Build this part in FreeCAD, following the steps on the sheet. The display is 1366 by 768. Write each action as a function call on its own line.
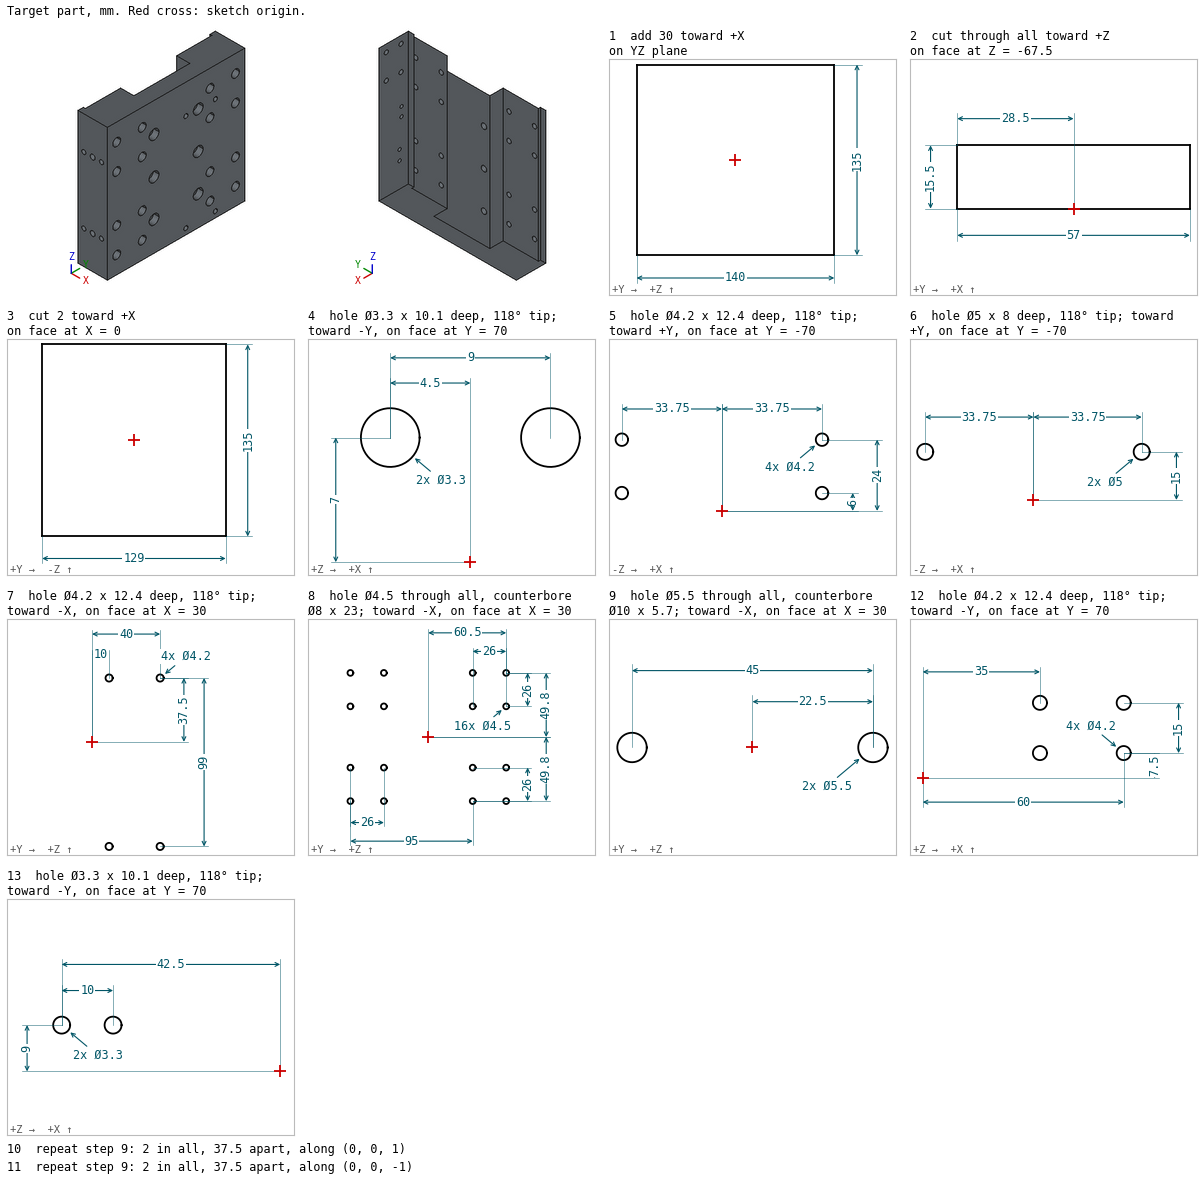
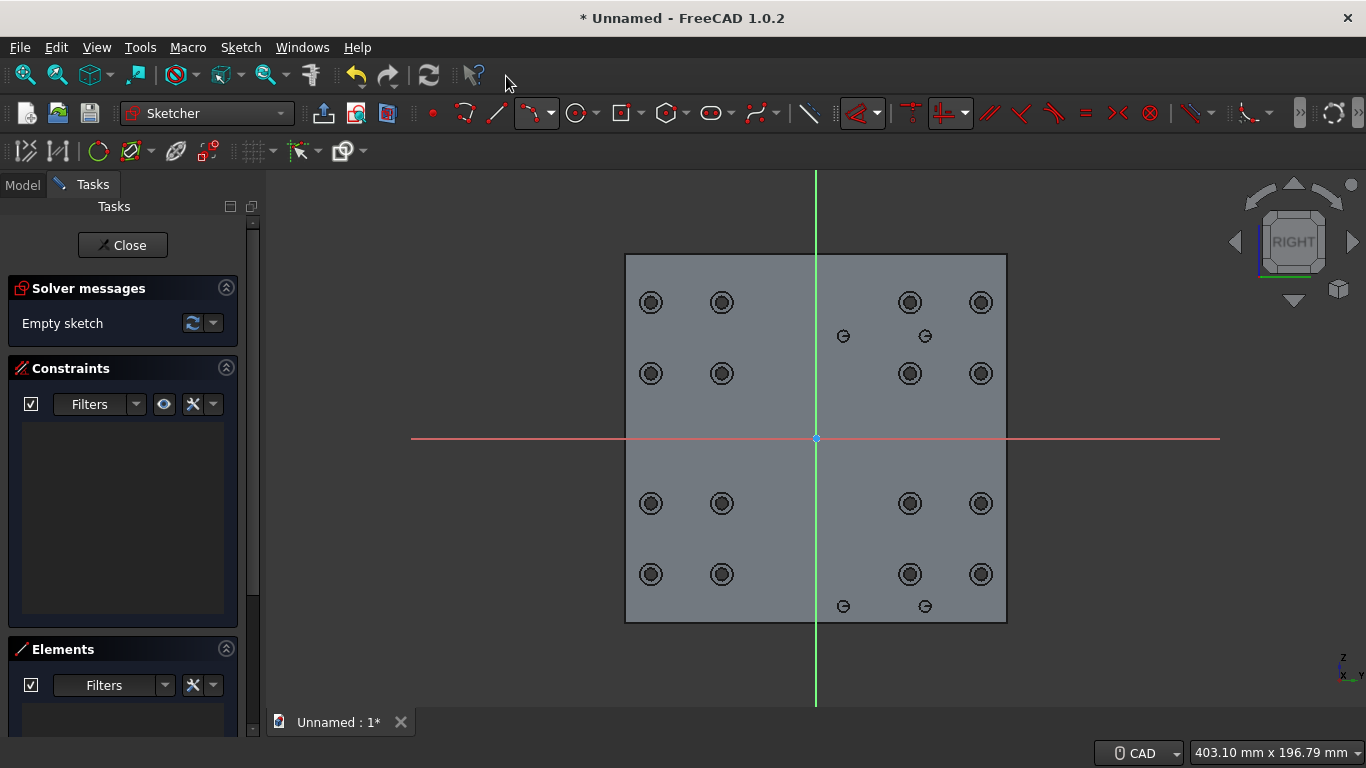
scroll(833, 439, up, 8)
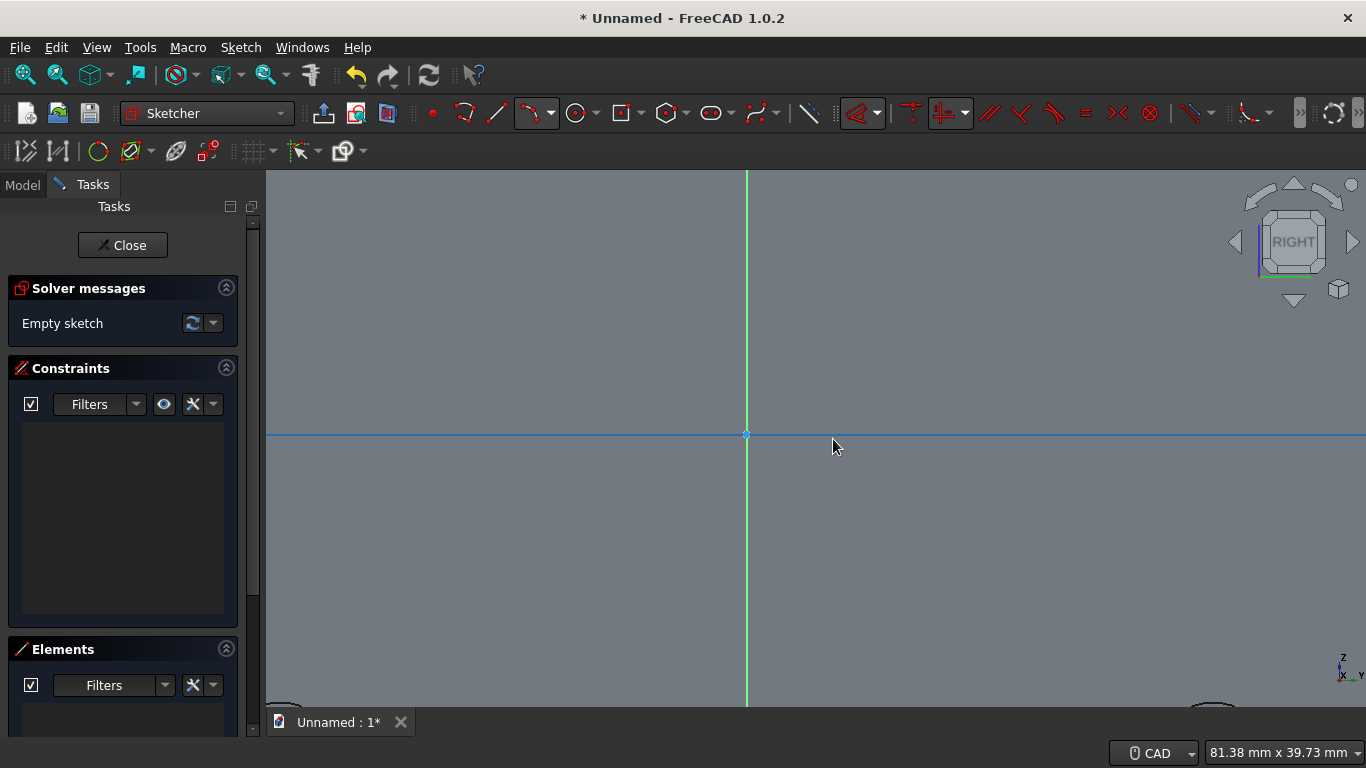
click(576, 114)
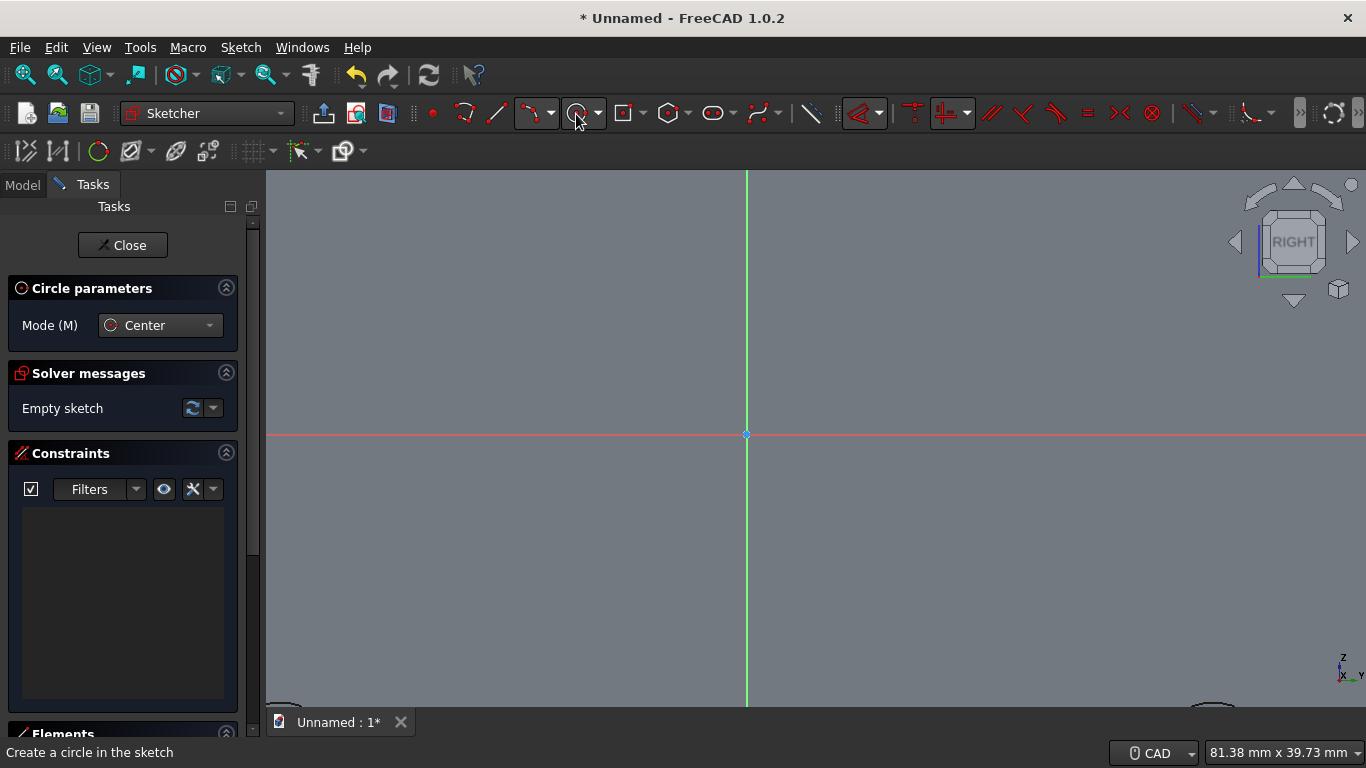
click(1051, 435)
click(1077, 408)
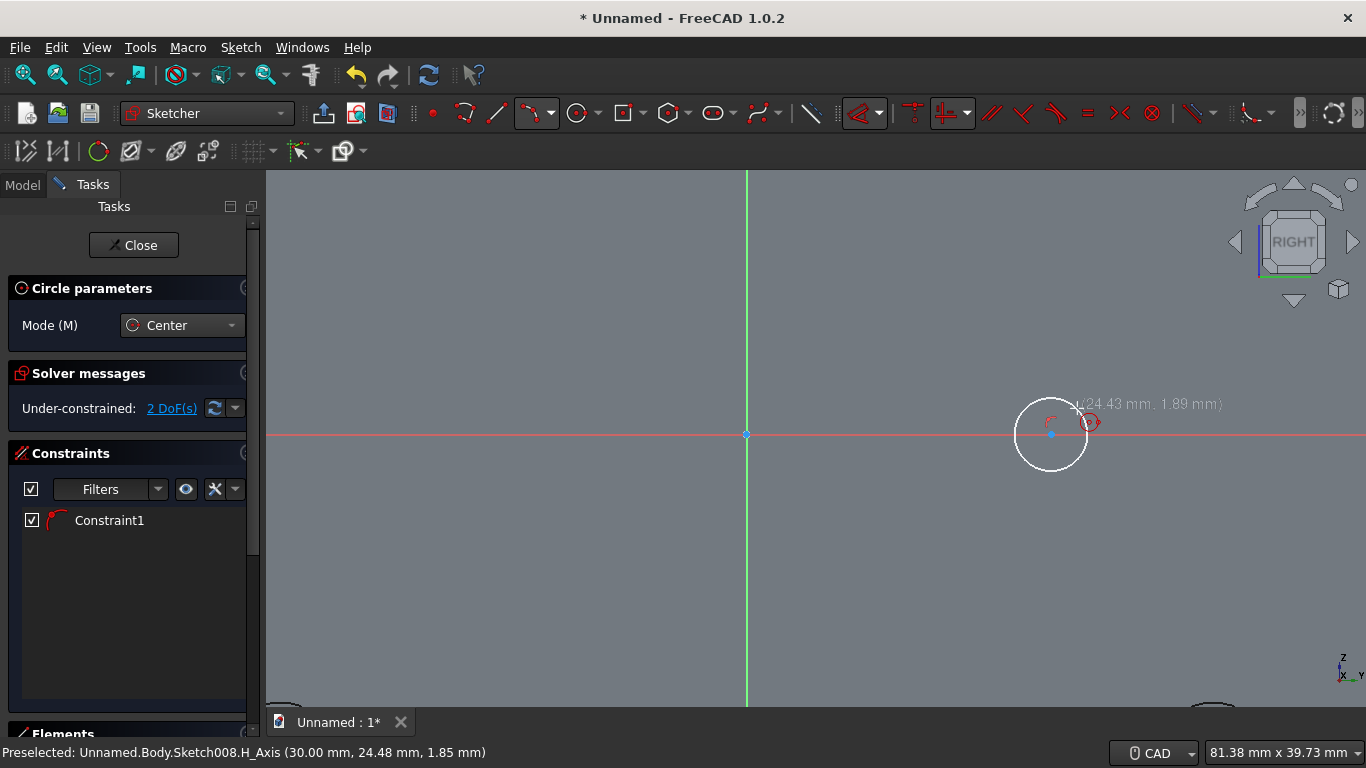
click(443, 435)
click(469, 408)
key(Escape)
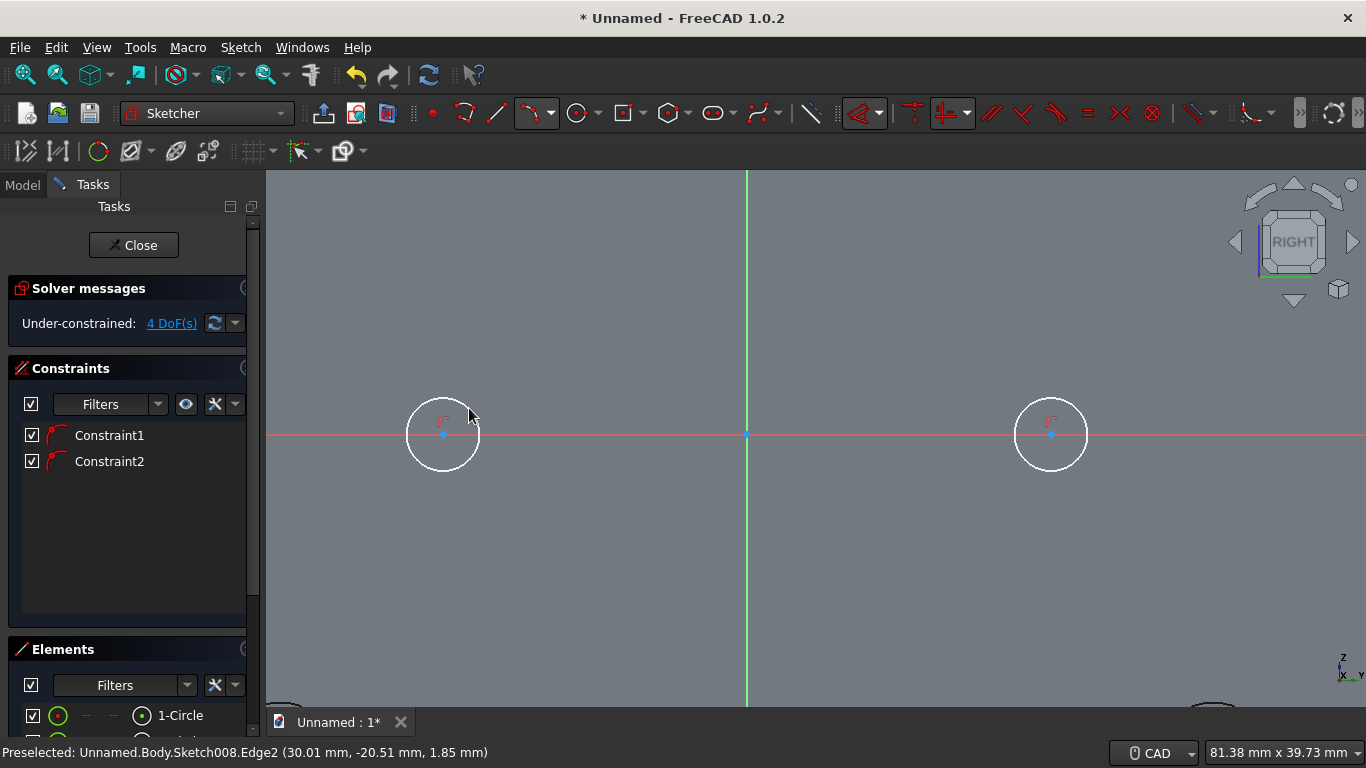
click(1077, 409)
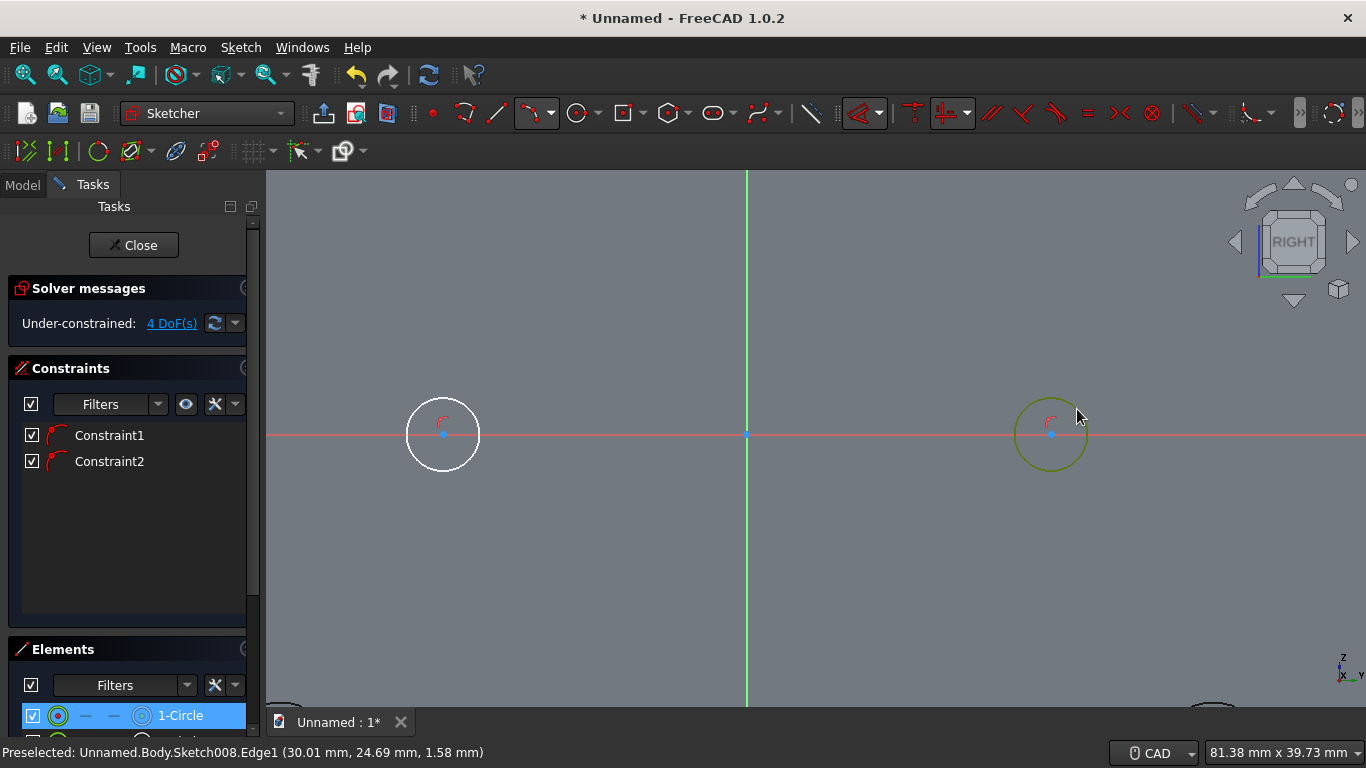
click(469, 409)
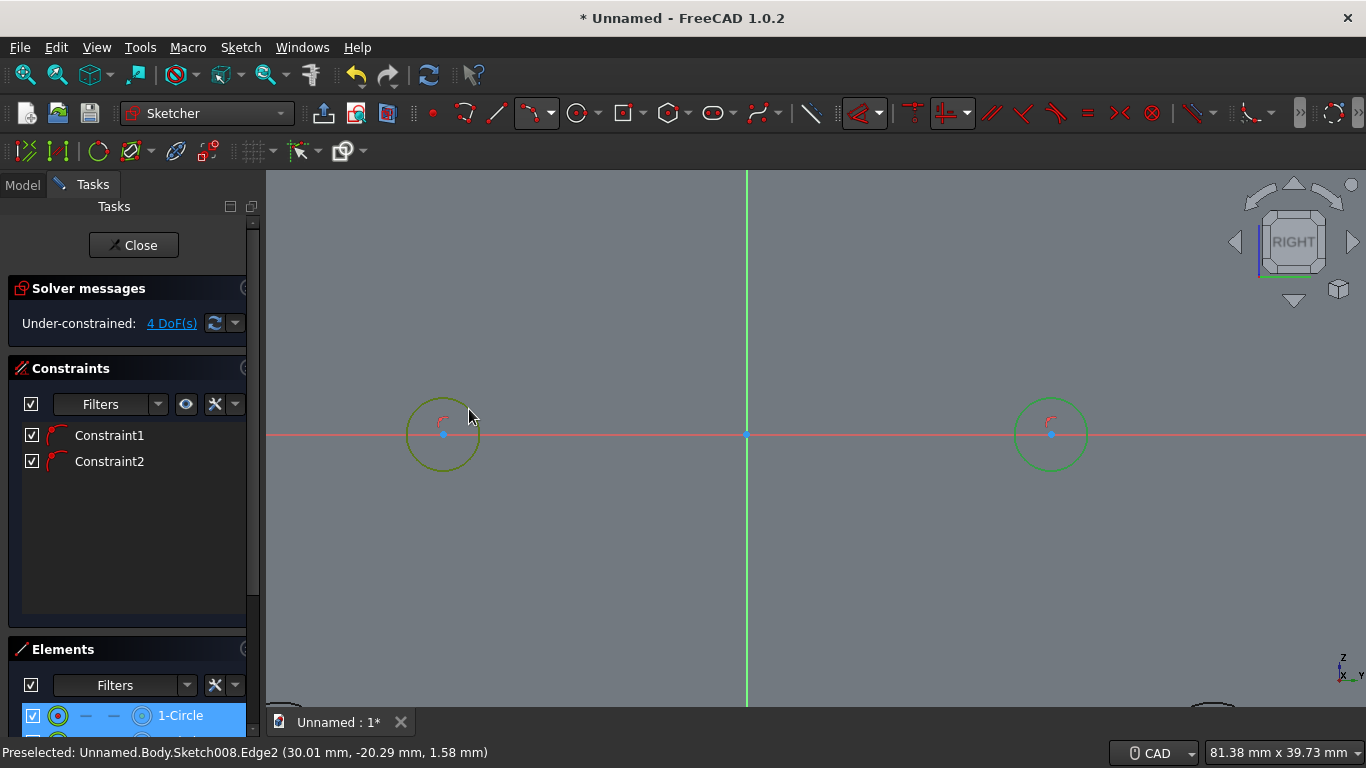
click(1088, 114)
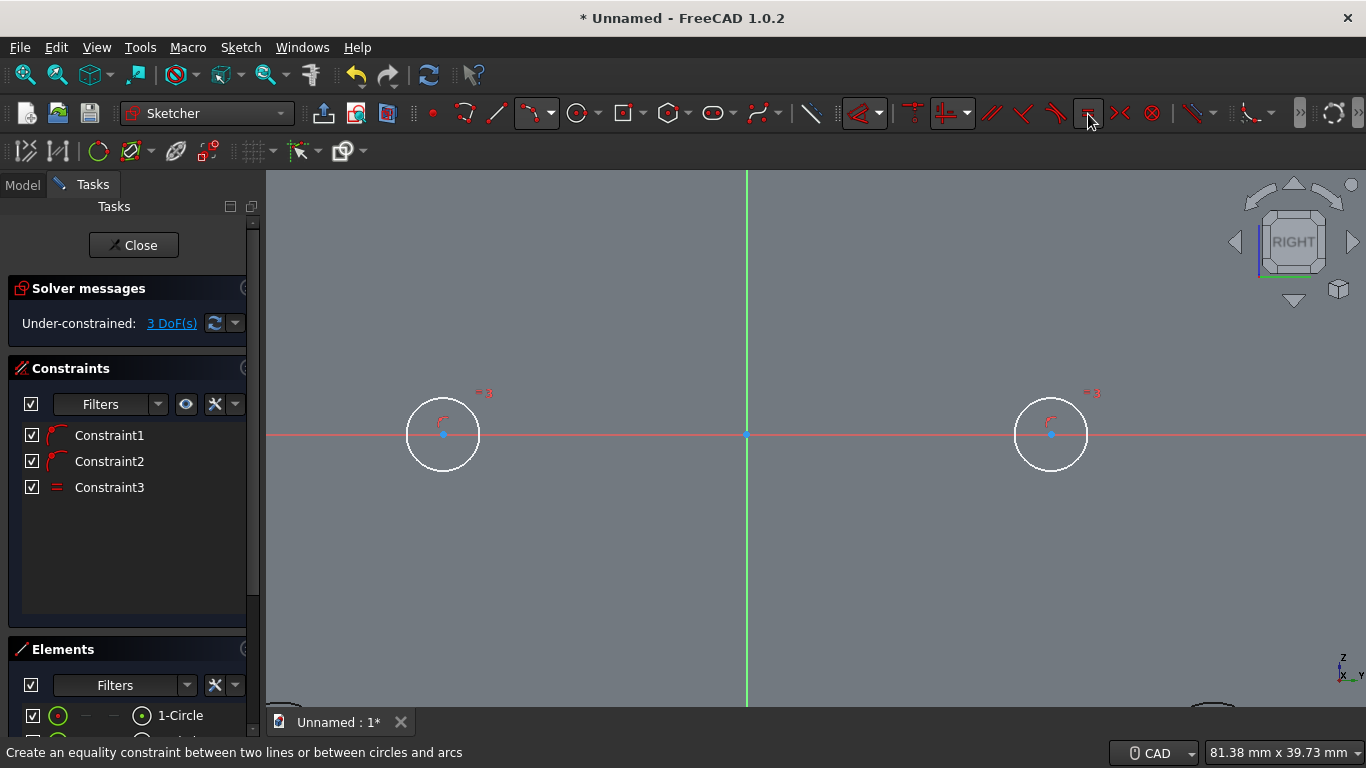
click(1077, 409)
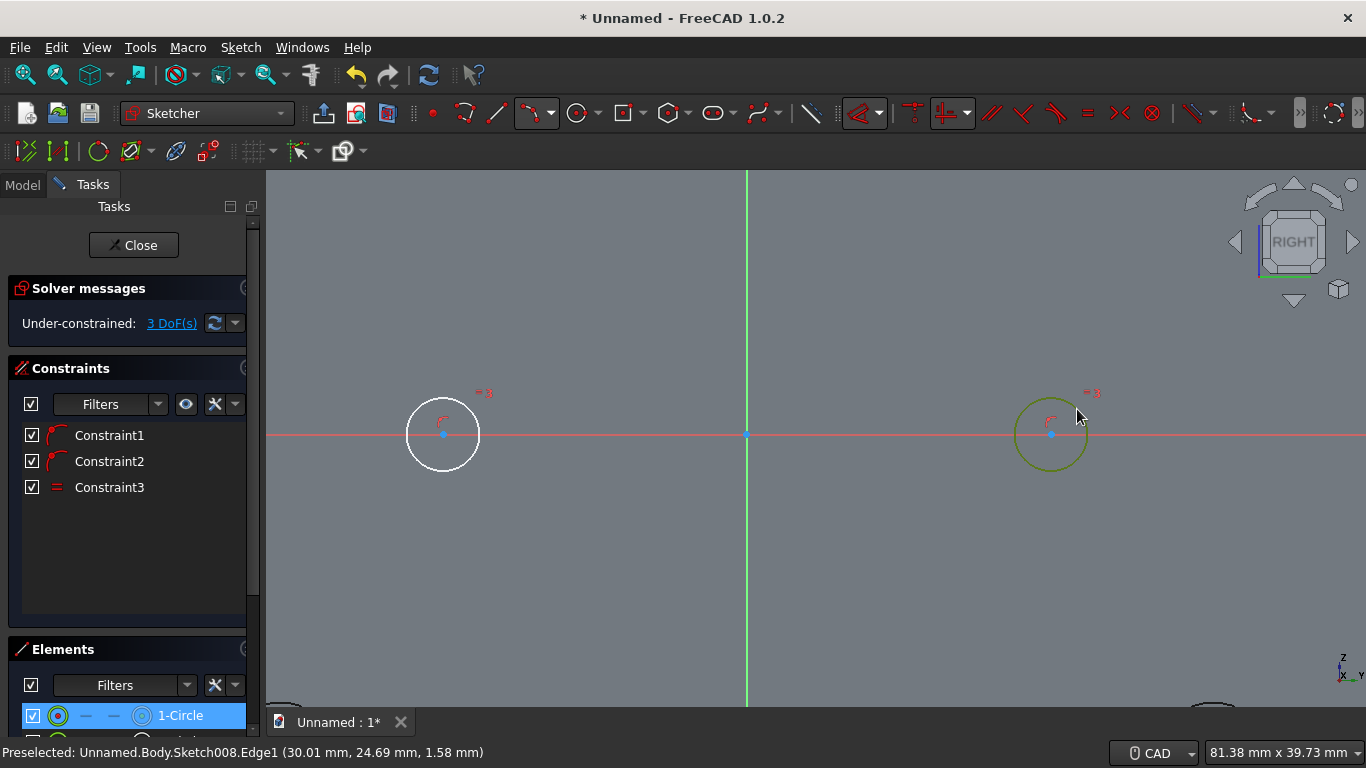
click(882, 114)